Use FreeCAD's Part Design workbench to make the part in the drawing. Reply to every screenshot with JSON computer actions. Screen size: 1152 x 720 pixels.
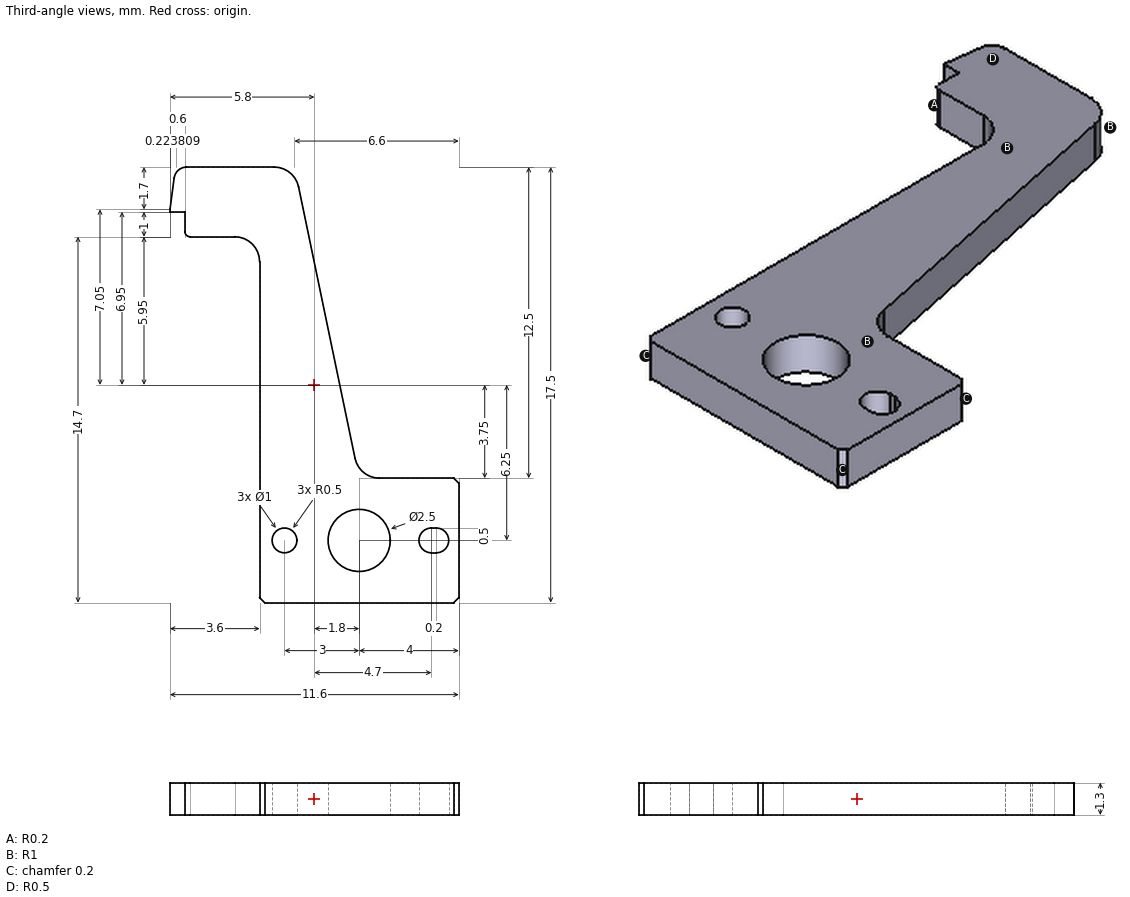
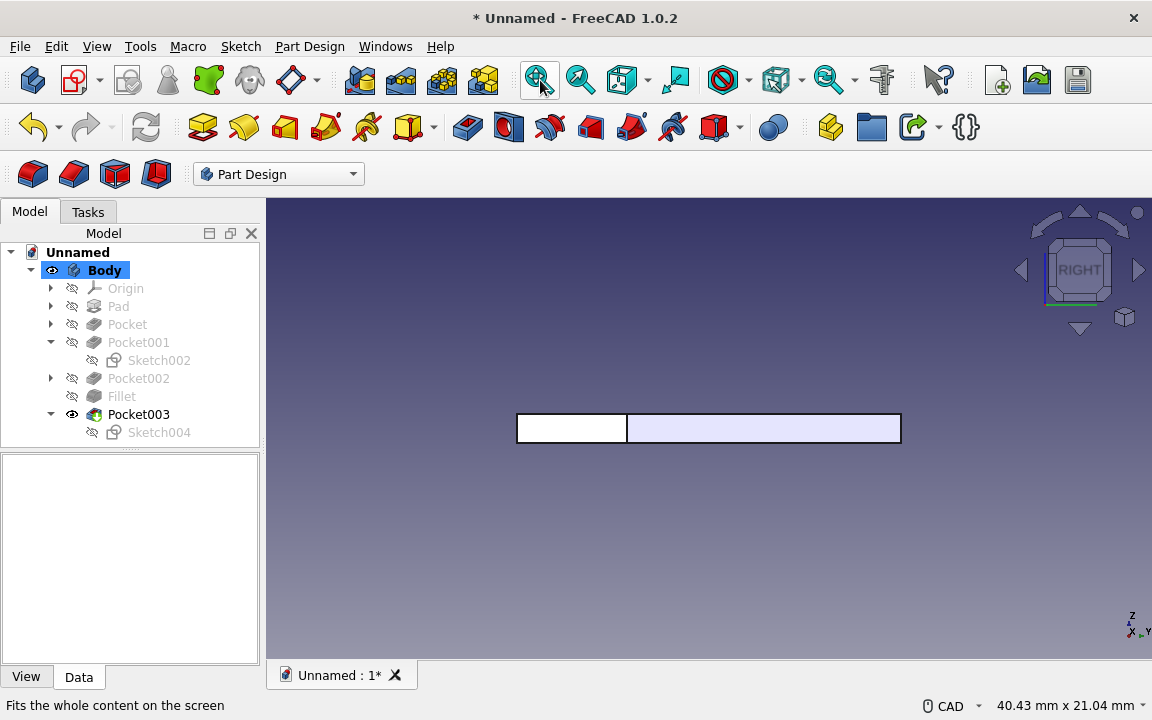
{"action": "key", "text": "v f"}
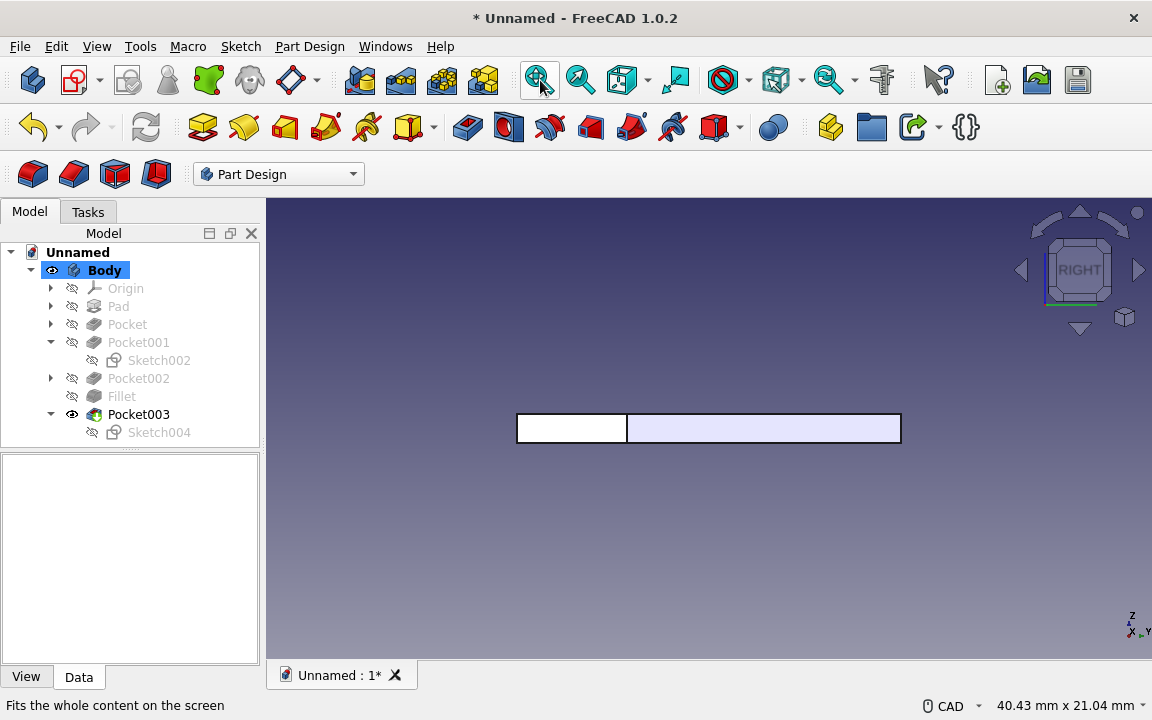
{"action": "key", "text": "5"}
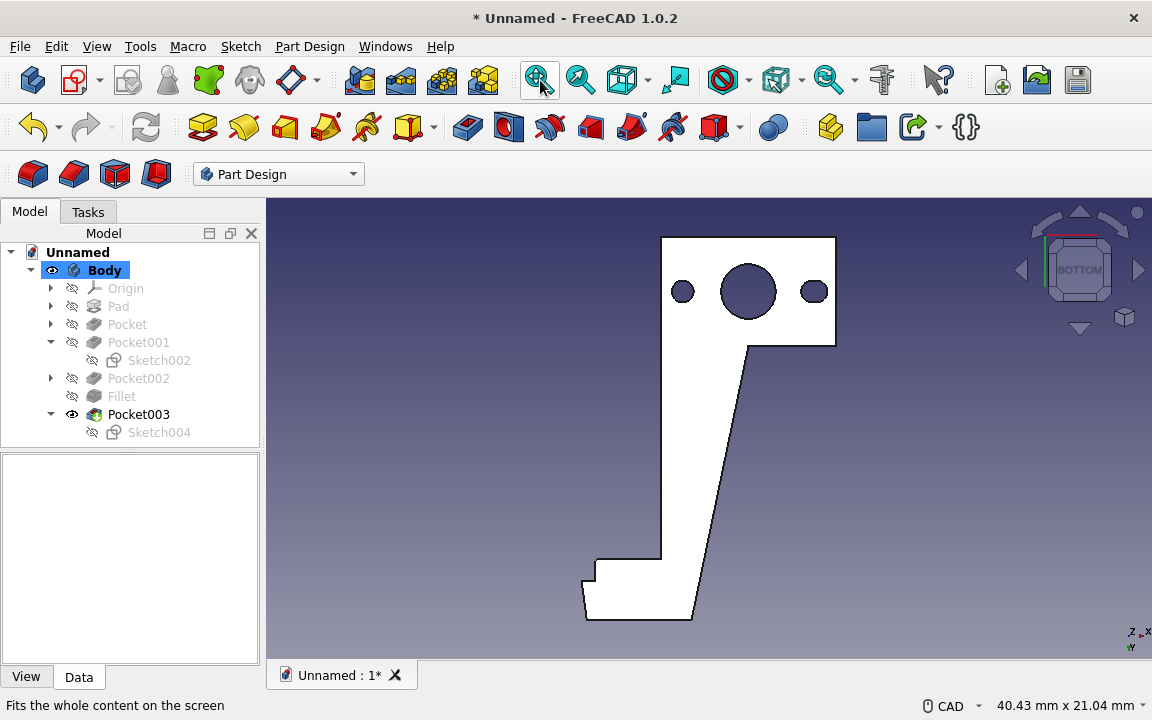
{"action": "key", "text": "4"}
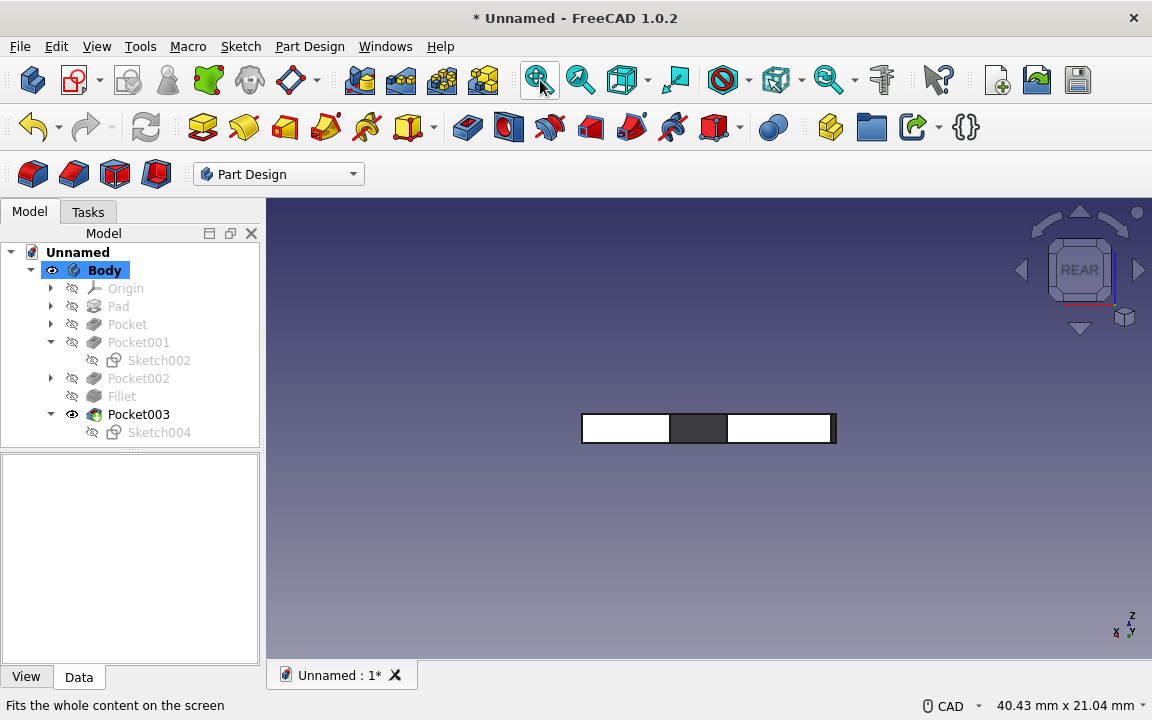
{"action": "key", "text": "v f"}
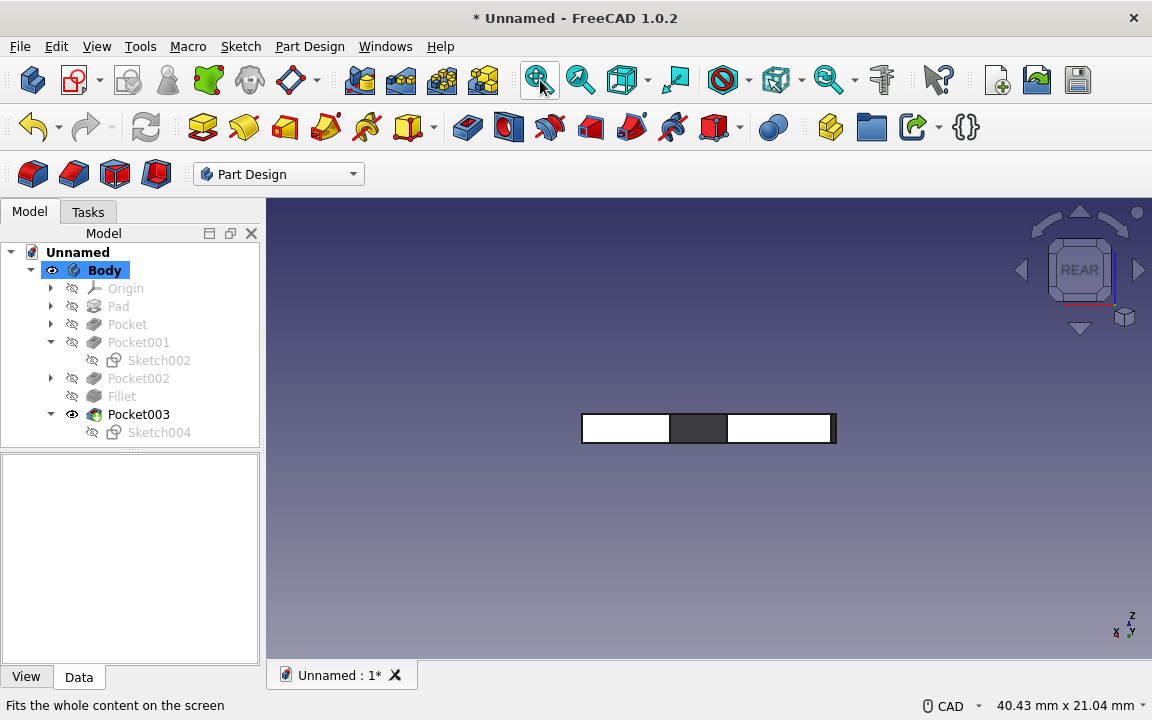
{"action": "left_click", "coordinate": [727, 428]}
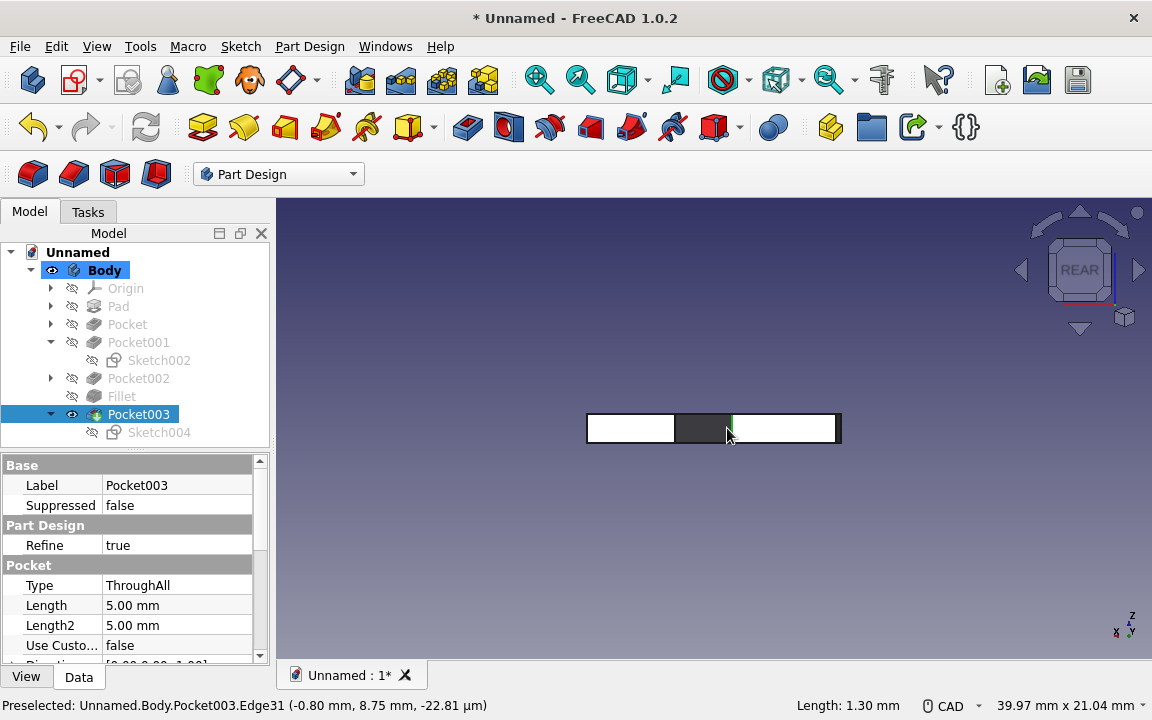
{"action": "key", "text": "6"}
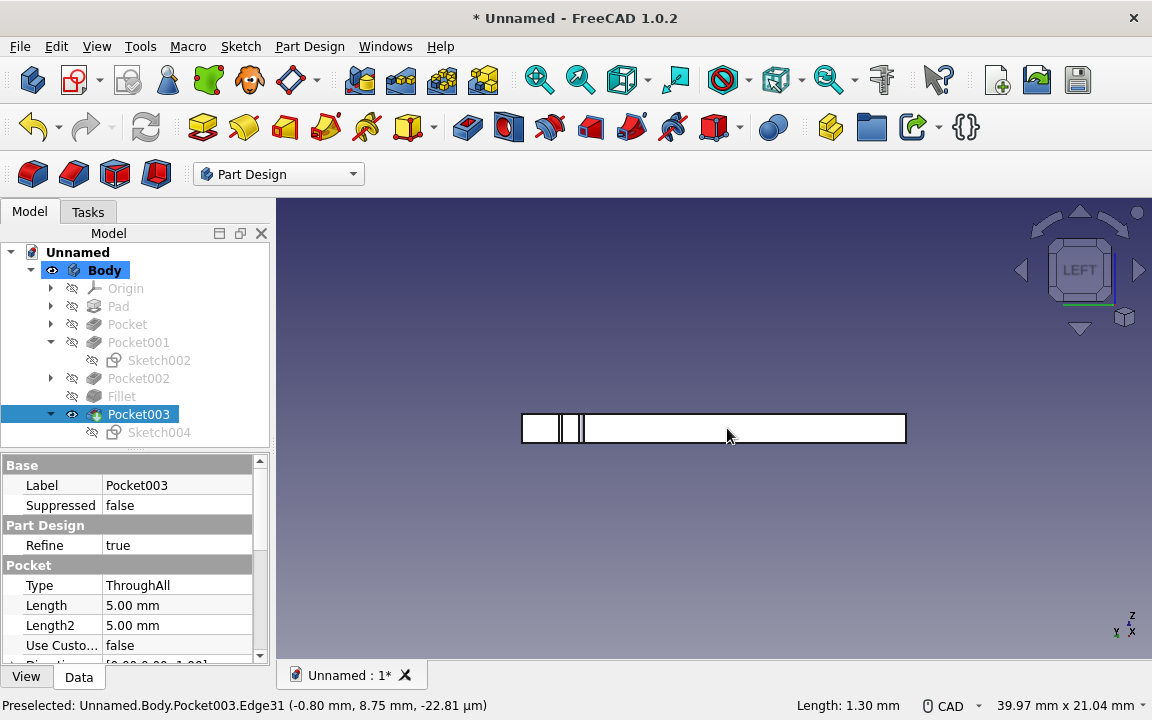
{"action": "left_click", "coordinate": [540, 80]}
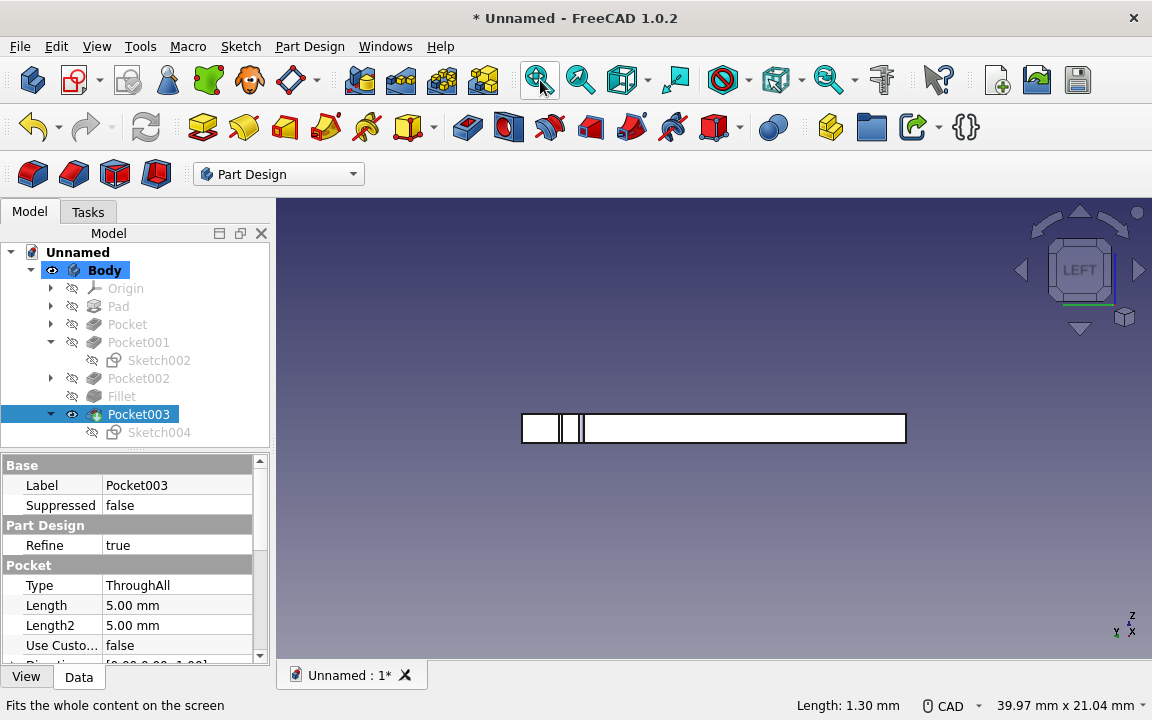
{"action": "key", "text": "v 3"}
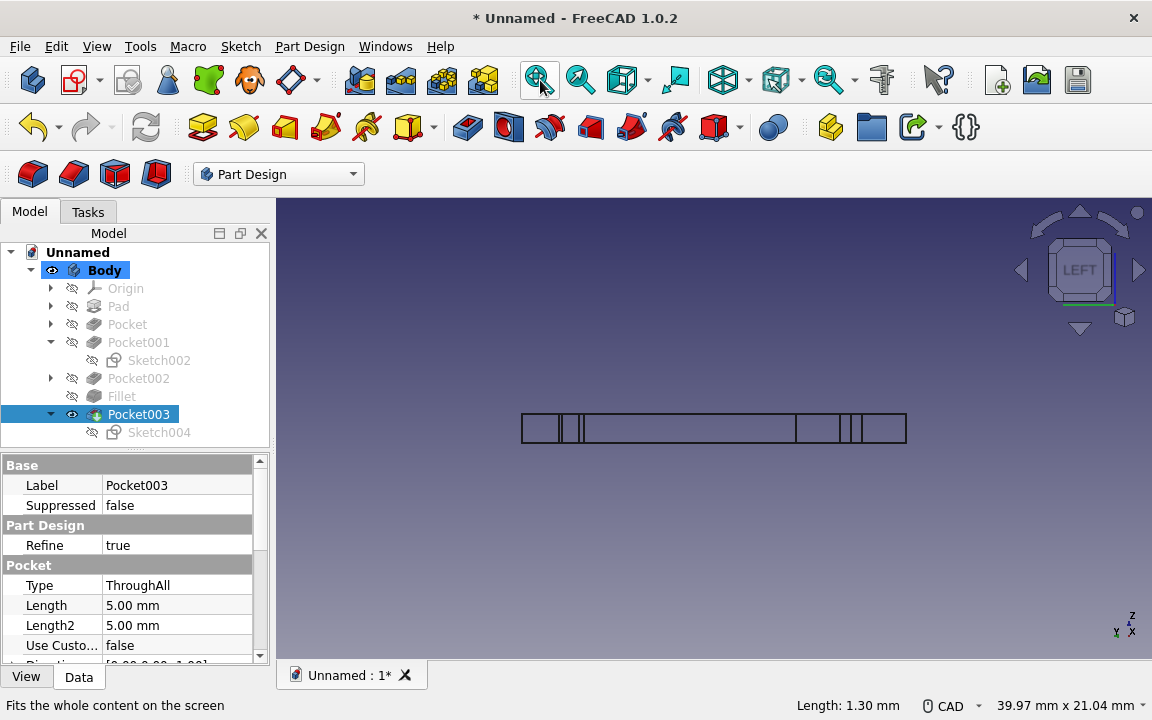
{"action": "key", "text": "0"}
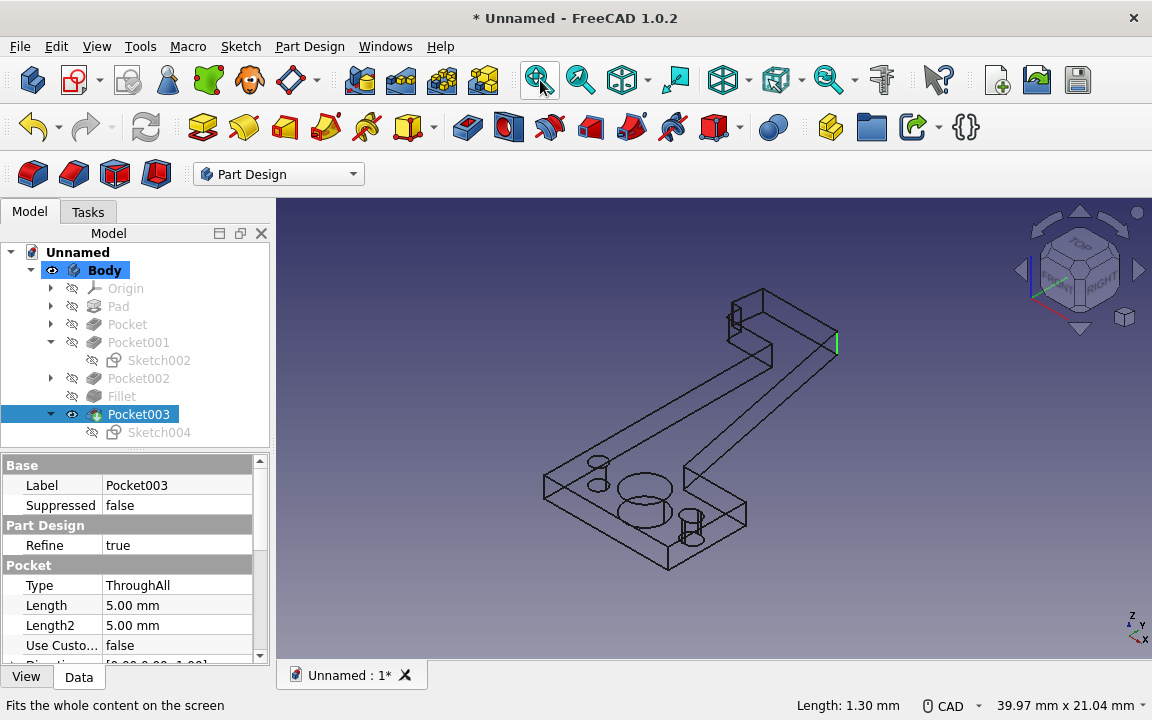
{"action": "left_click", "coordinate": [772, 355], "text": "ctrl"}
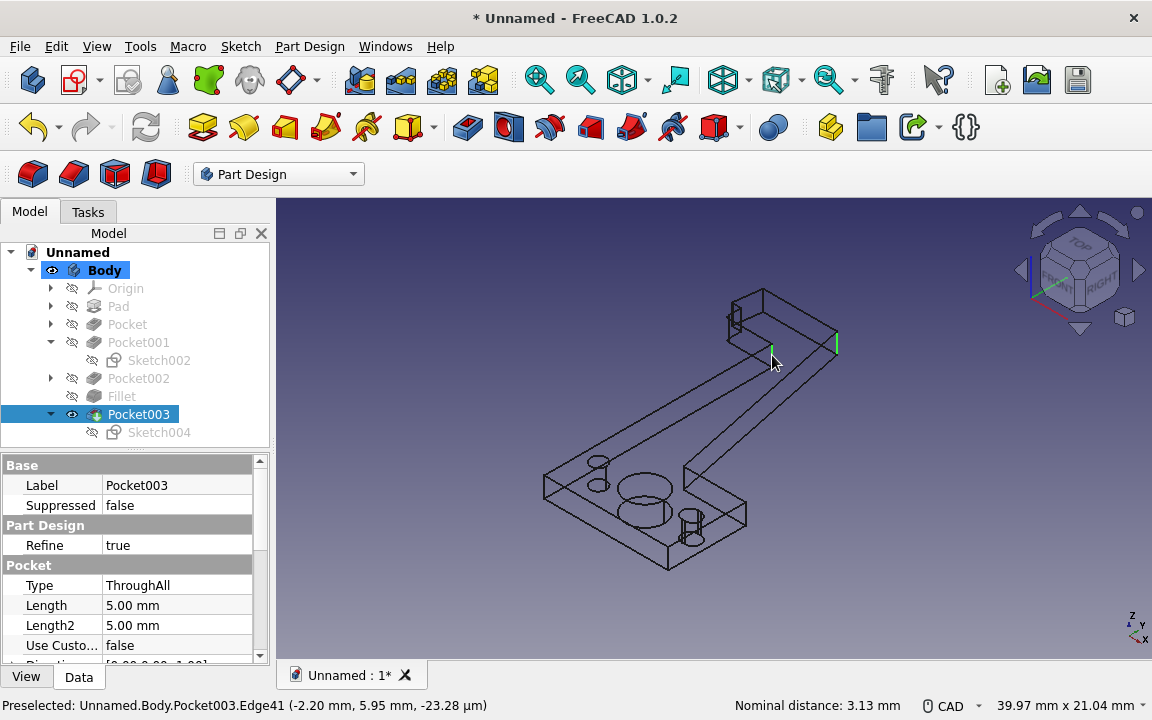
{"action": "left_click", "coordinate": [684, 477], "text": "ctrl"}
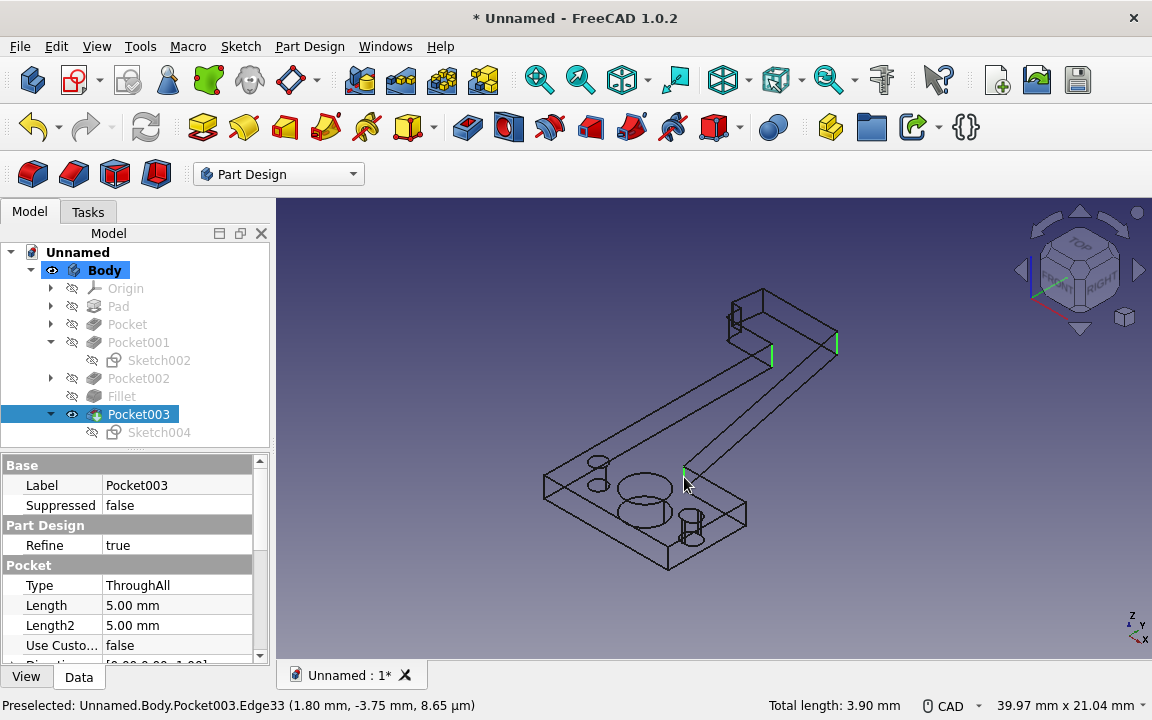
{"action": "key", "text": "v 1"}